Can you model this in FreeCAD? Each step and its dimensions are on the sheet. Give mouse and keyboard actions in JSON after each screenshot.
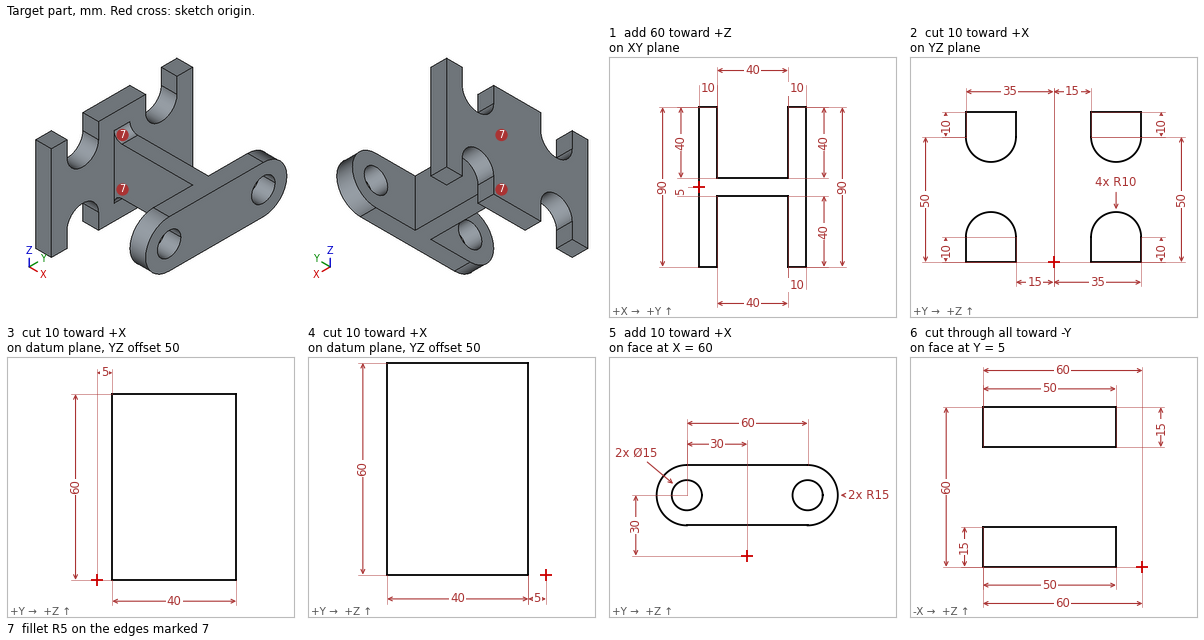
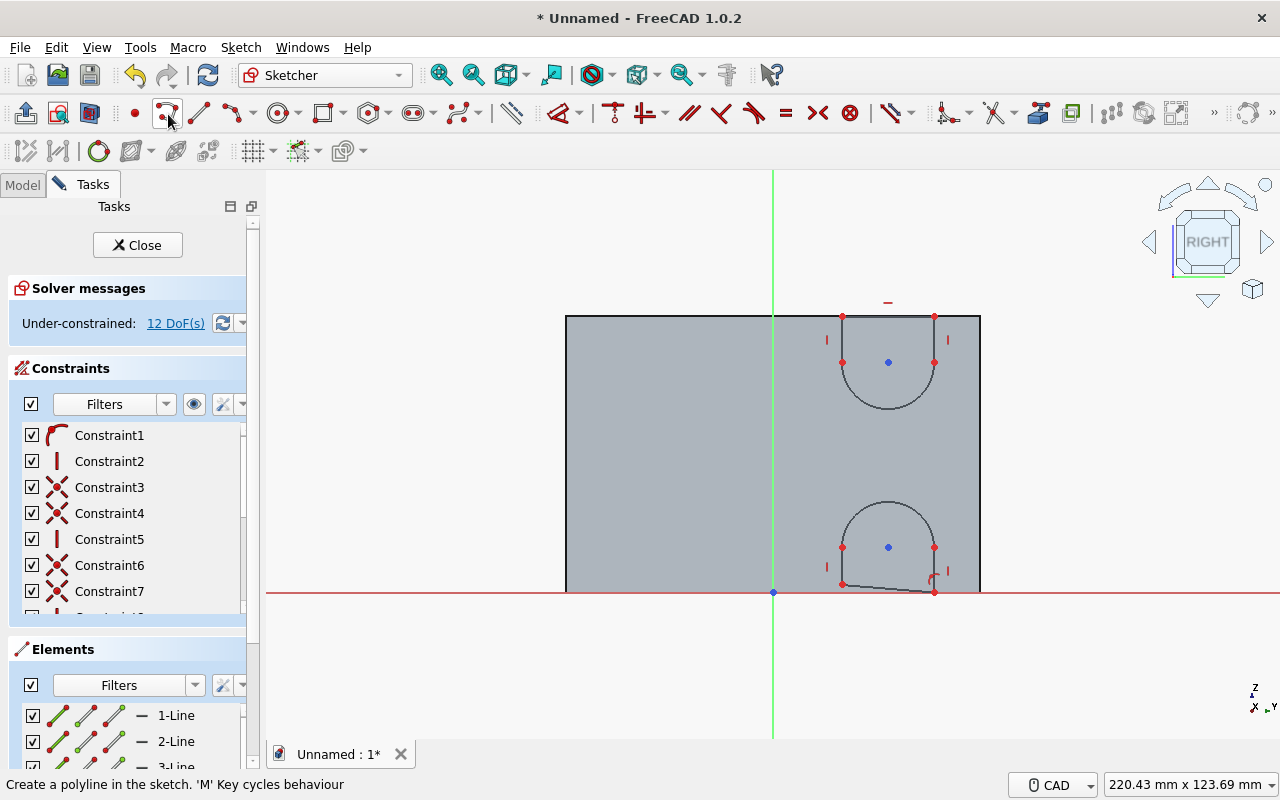
{"action": "left_click", "coordinate": [704, 547]}
{"action": "left_click", "coordinate": [704, 593]}
{"action": "left_click", "coordinate": [612, 584]}
{"action": "left_click", "coordinate": [612, 547]}
{"action": "right_click", "coordinate": [612, 547]}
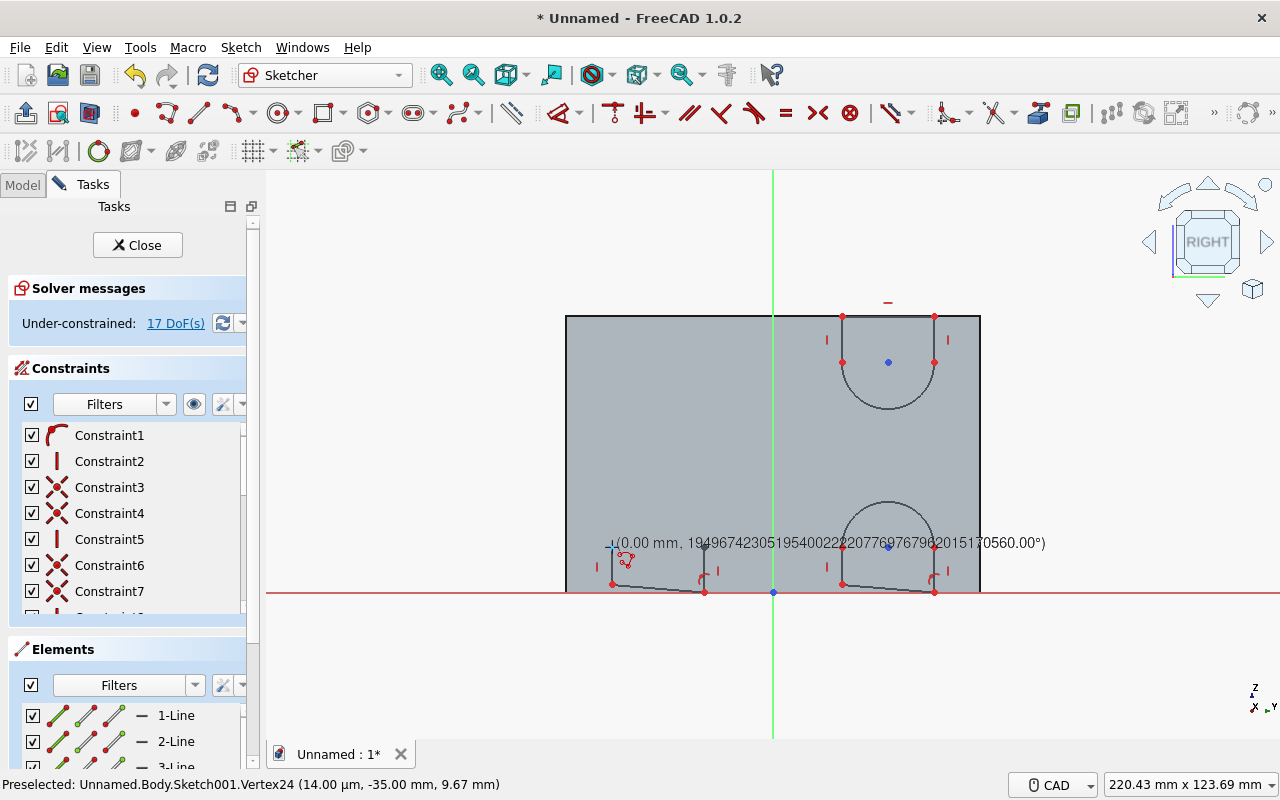
{"action": "left_click", "coordinate": [232, 114]}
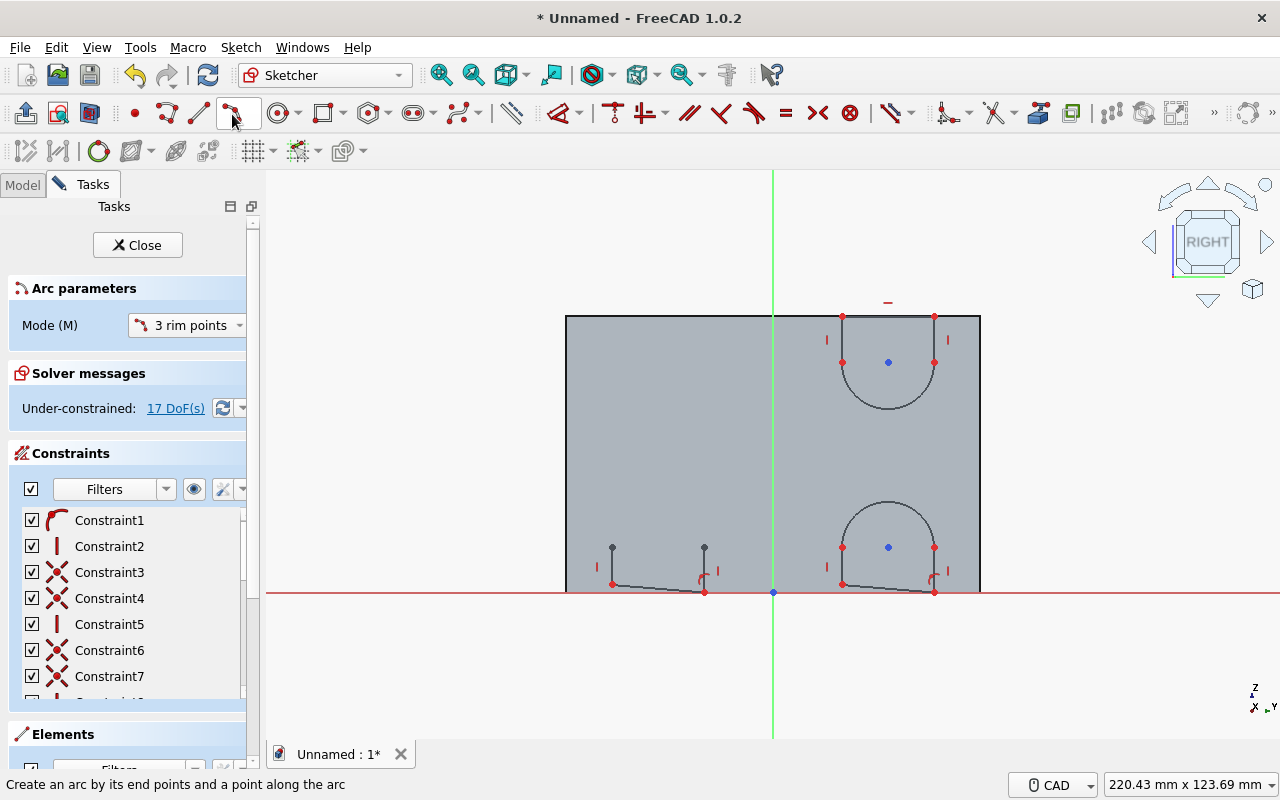
{"action": "left_click", "coordinate": [612, 548]}
{"action": "left_click", "coordinate": [704, 548]}
{"action": "left_click", "coordinate": [658, 501]}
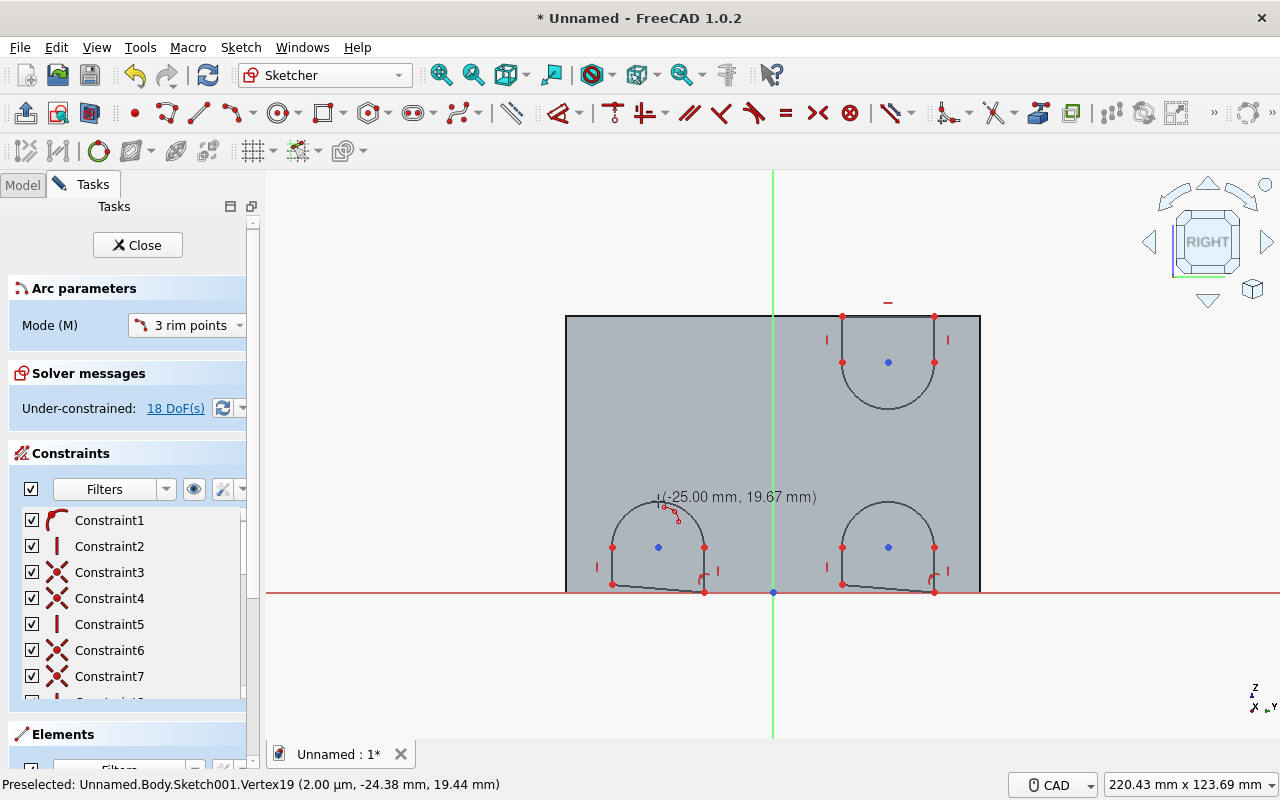
{"action": "left_click", "coordinate": [168, 114]}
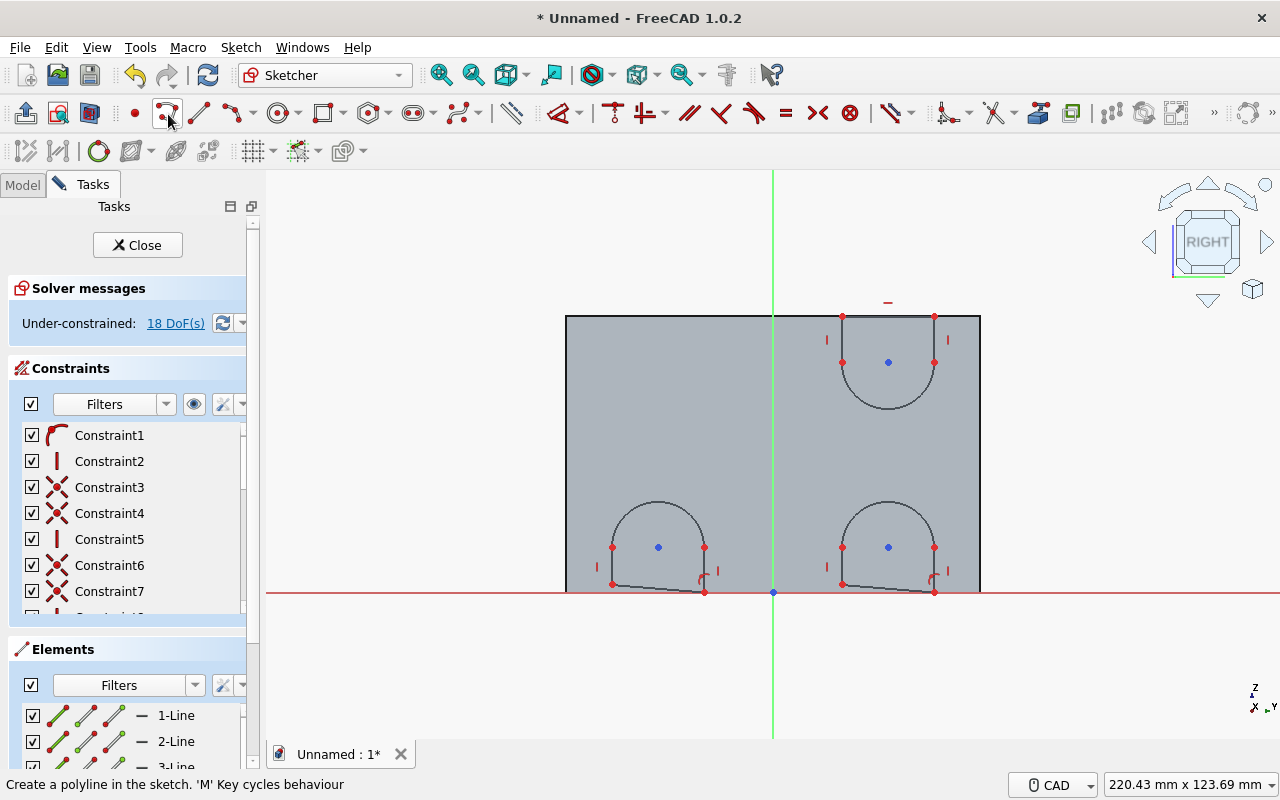
{"action": "left_click", "coordinate": [612, 362]}
{"action": "left_click", "coordinate": [612, 316]}
{"action": "left_click", "coordinate": [704, 316]}
{"action": "left_click", "coordinate": [704, 362]}
{"action": "right_click", "coordinate": [704, 362]}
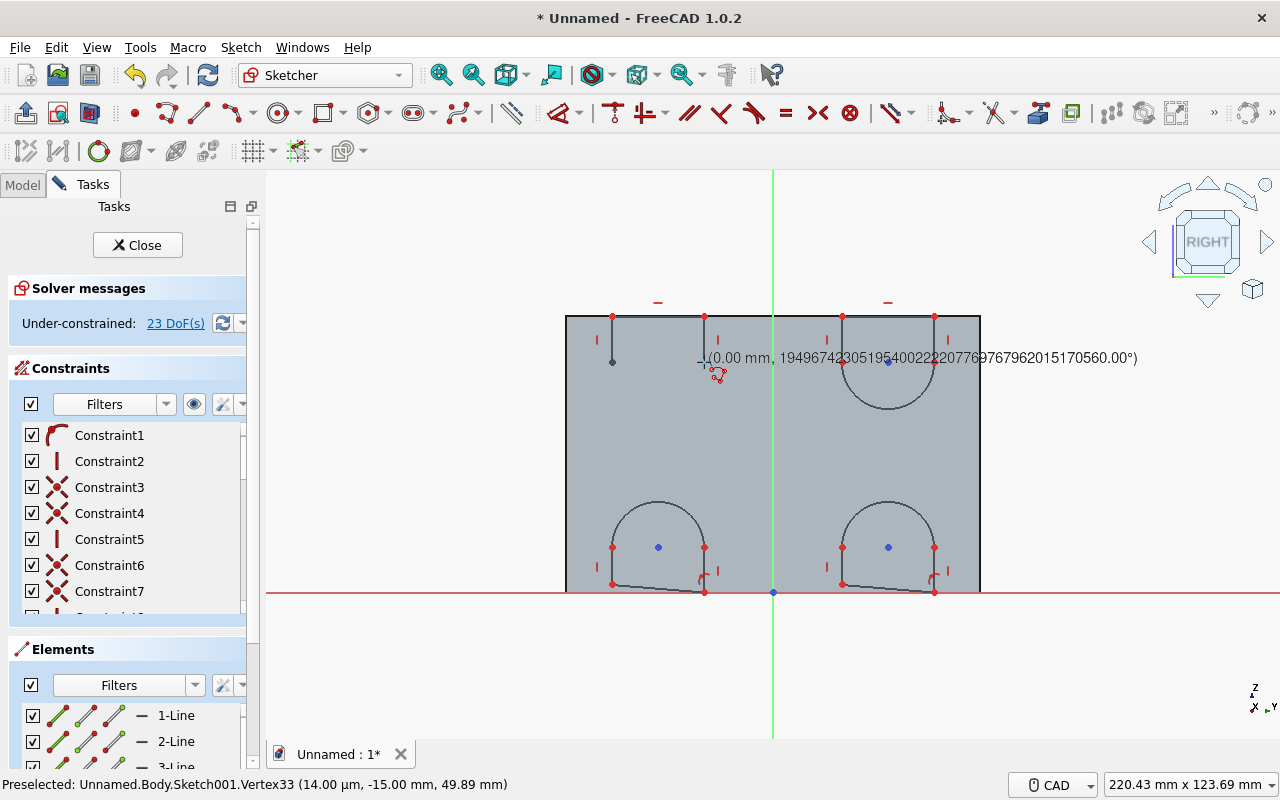
{"action": "left_click", "coordinate": [232, 114]}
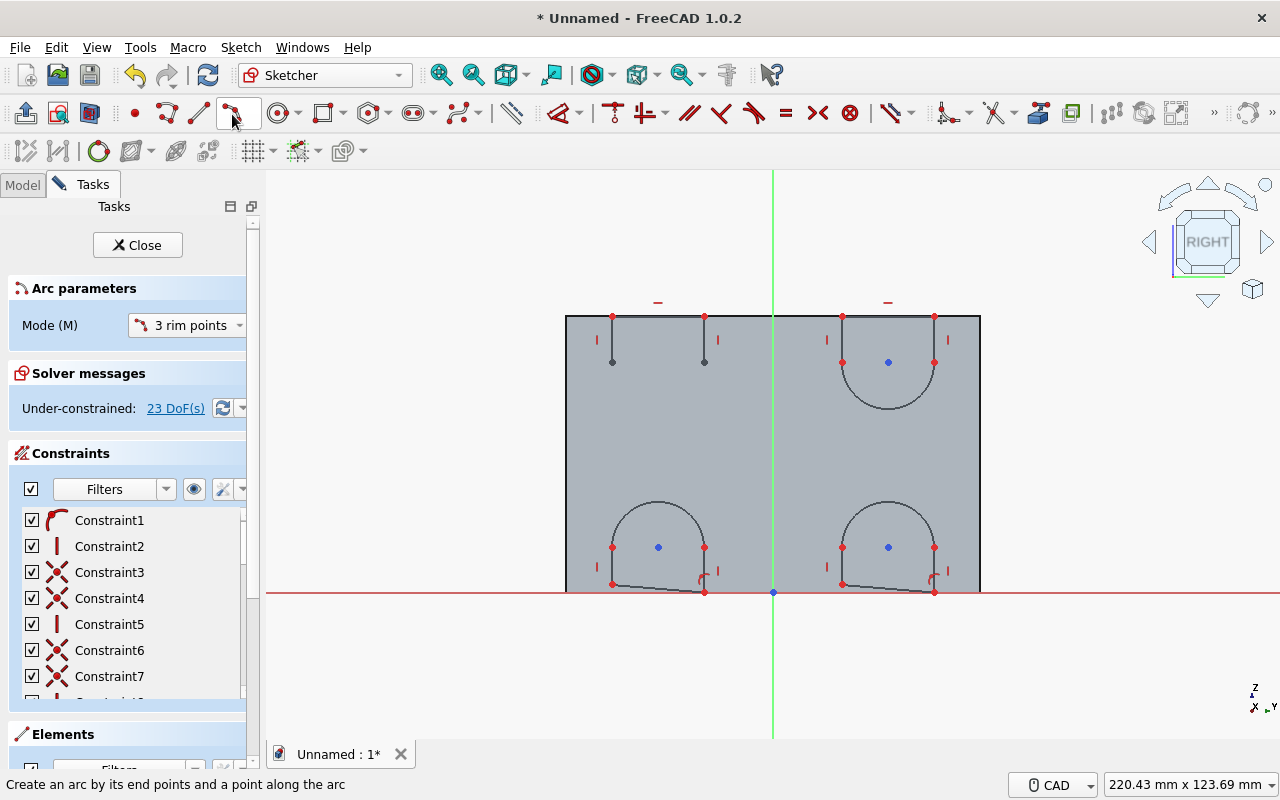
{"action": "left_click", "coordinate": [704, 363]}
{"action": "left_click", "coordinate": [612, 363]}
{"action": "left_click", "coordinate": [658, 408]}
{"action": "key", "text": "Escape"}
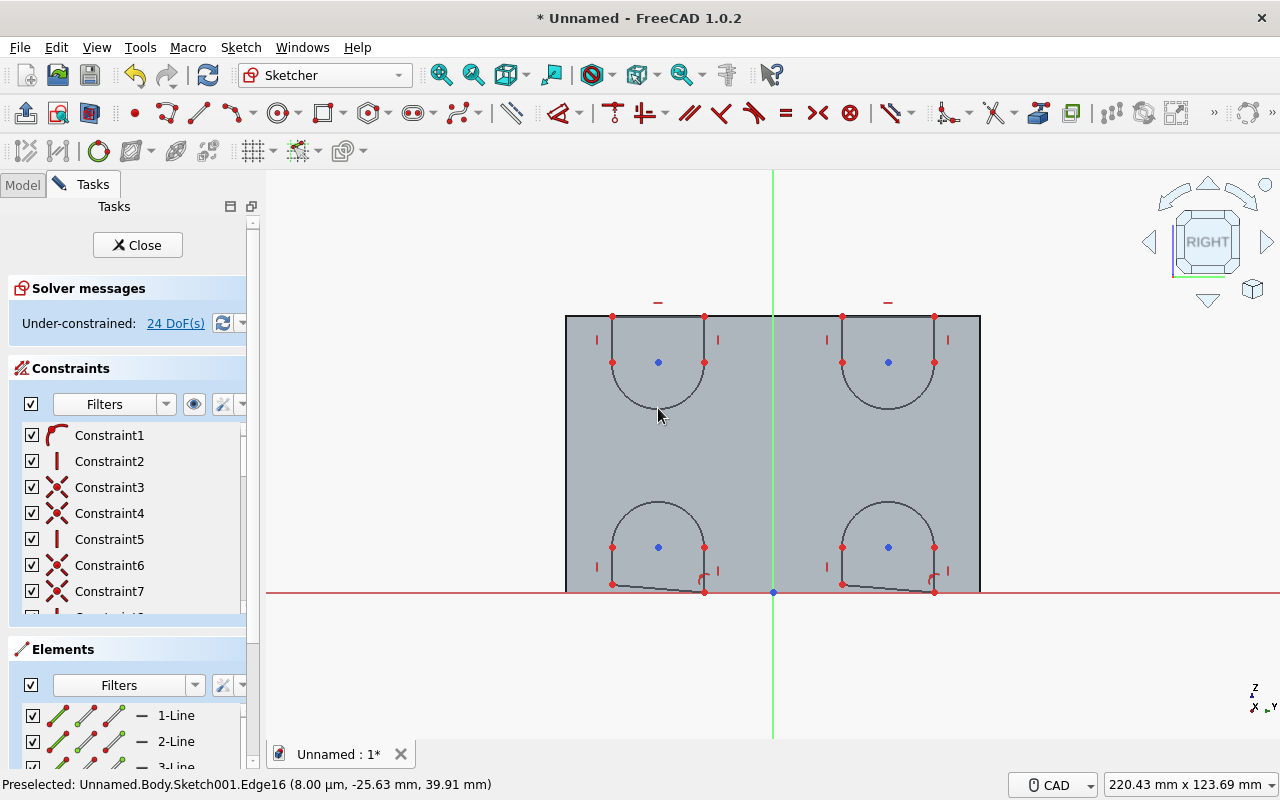
{"action": "left_click", "coordinate": [934, 561]}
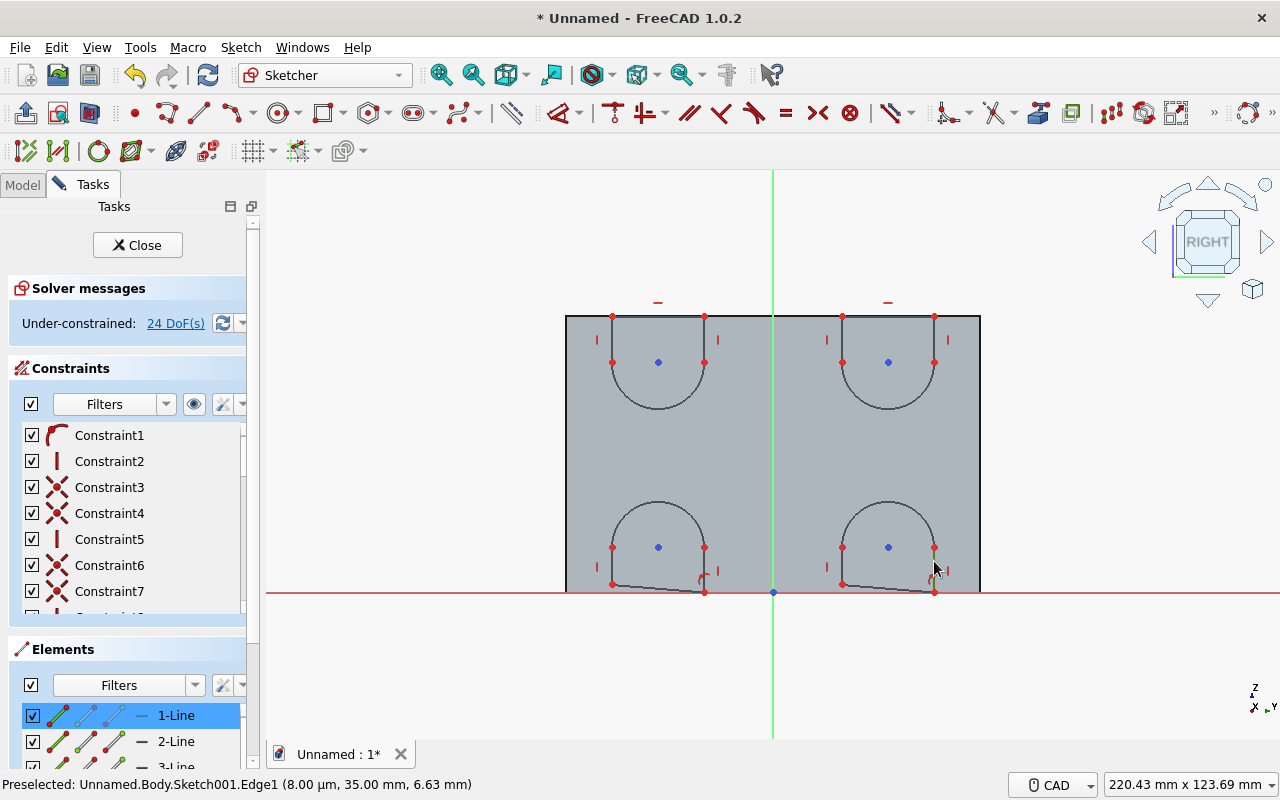
{"action": "left_click", "coordinate": [915, 511]}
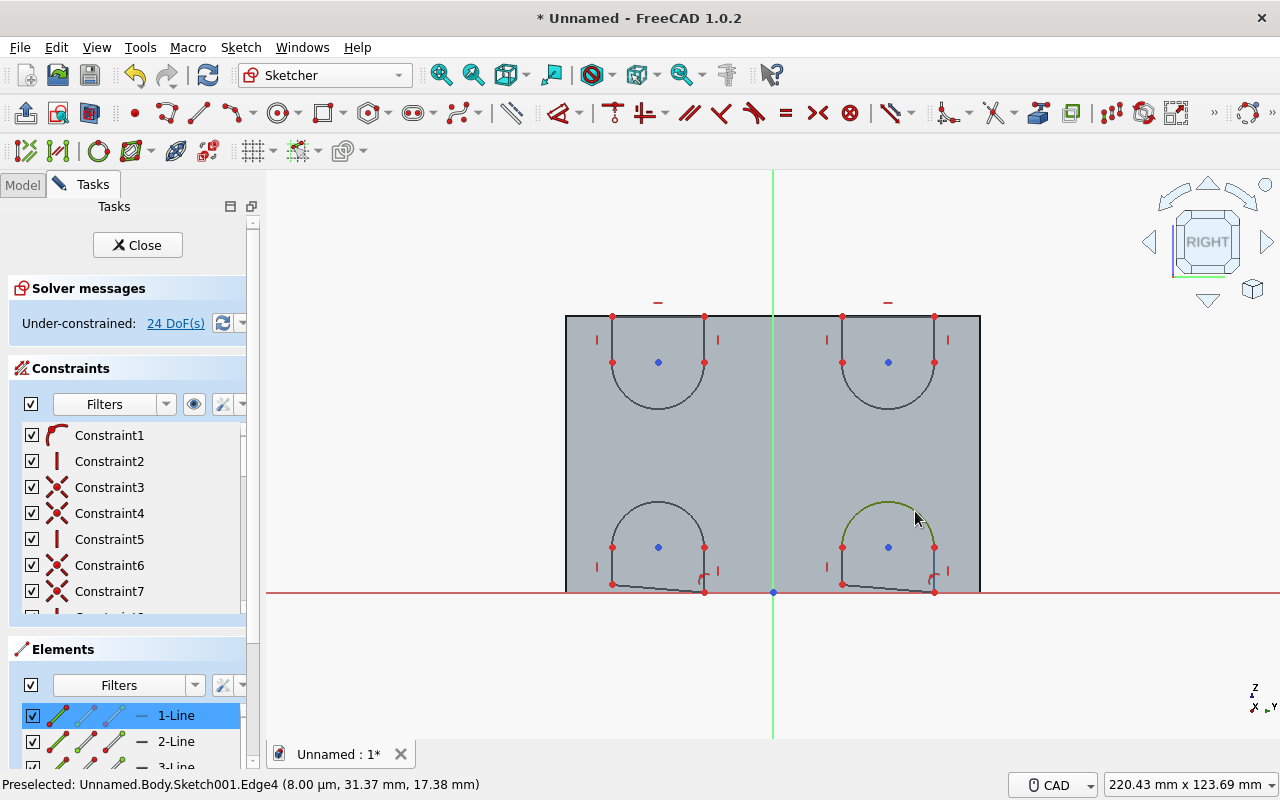
{"action": "left_click", "coordinate": [754, 114]}